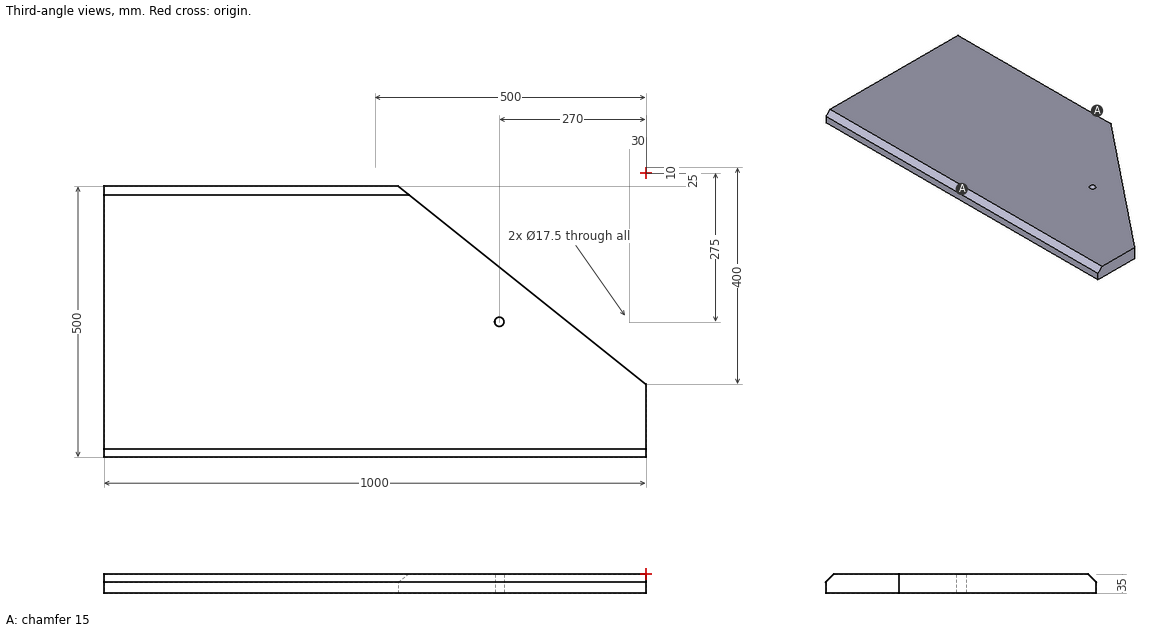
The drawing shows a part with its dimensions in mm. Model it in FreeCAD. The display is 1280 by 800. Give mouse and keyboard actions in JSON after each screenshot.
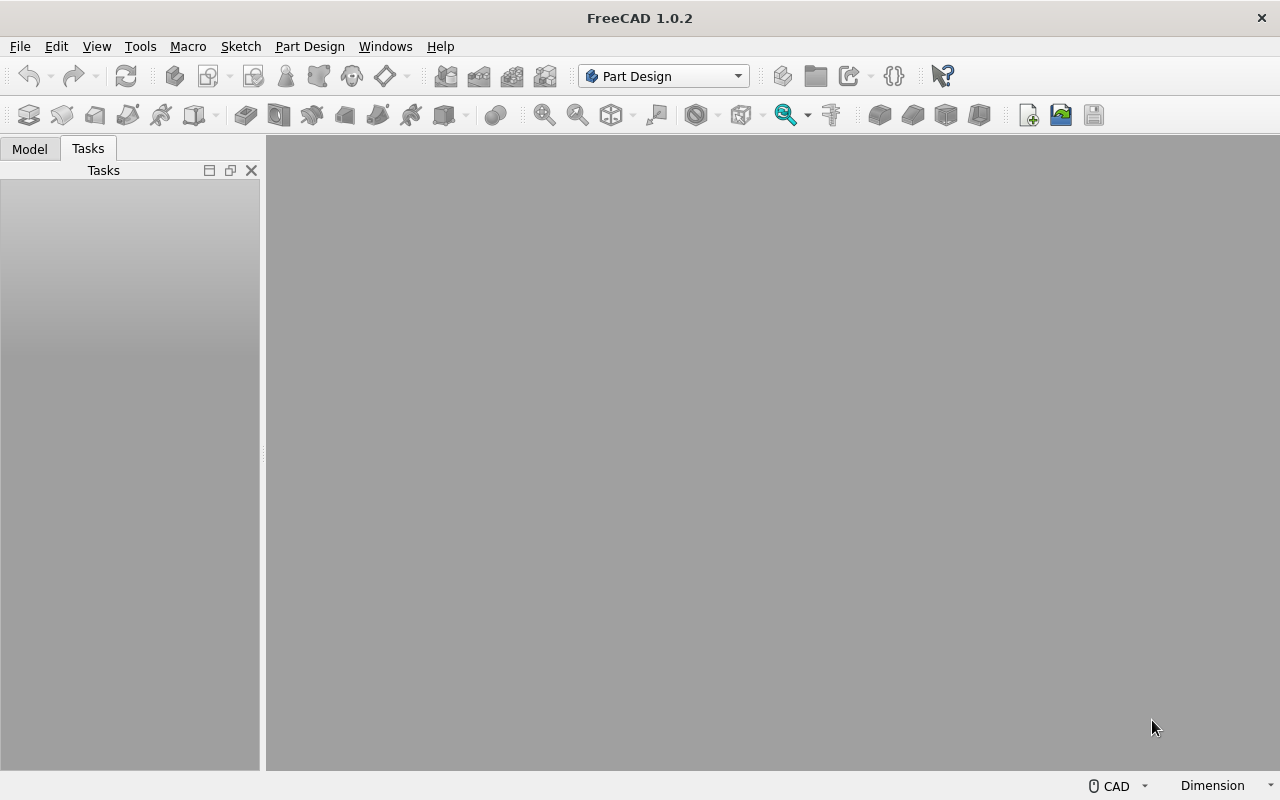
{"action": "key", "text": "ctrl+n"}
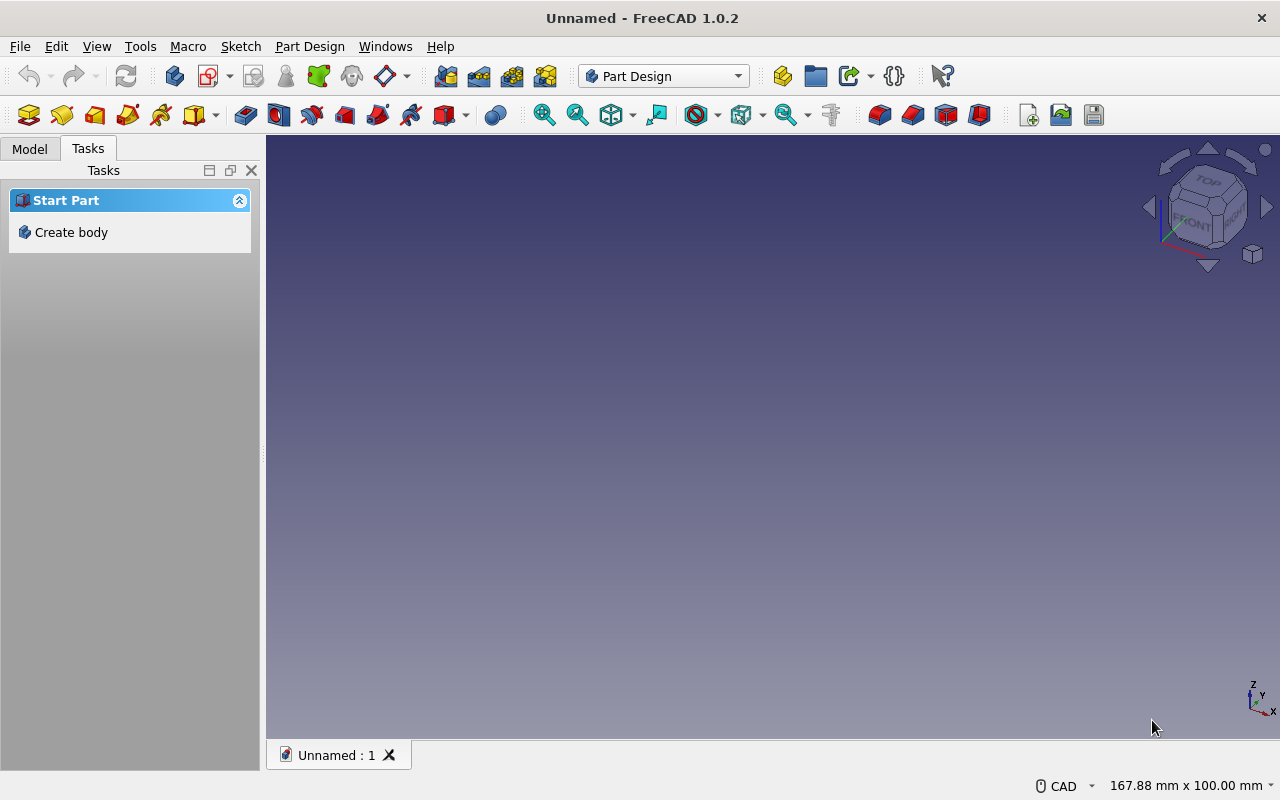
{"action": "left_click", "coordinate": [208, 76]}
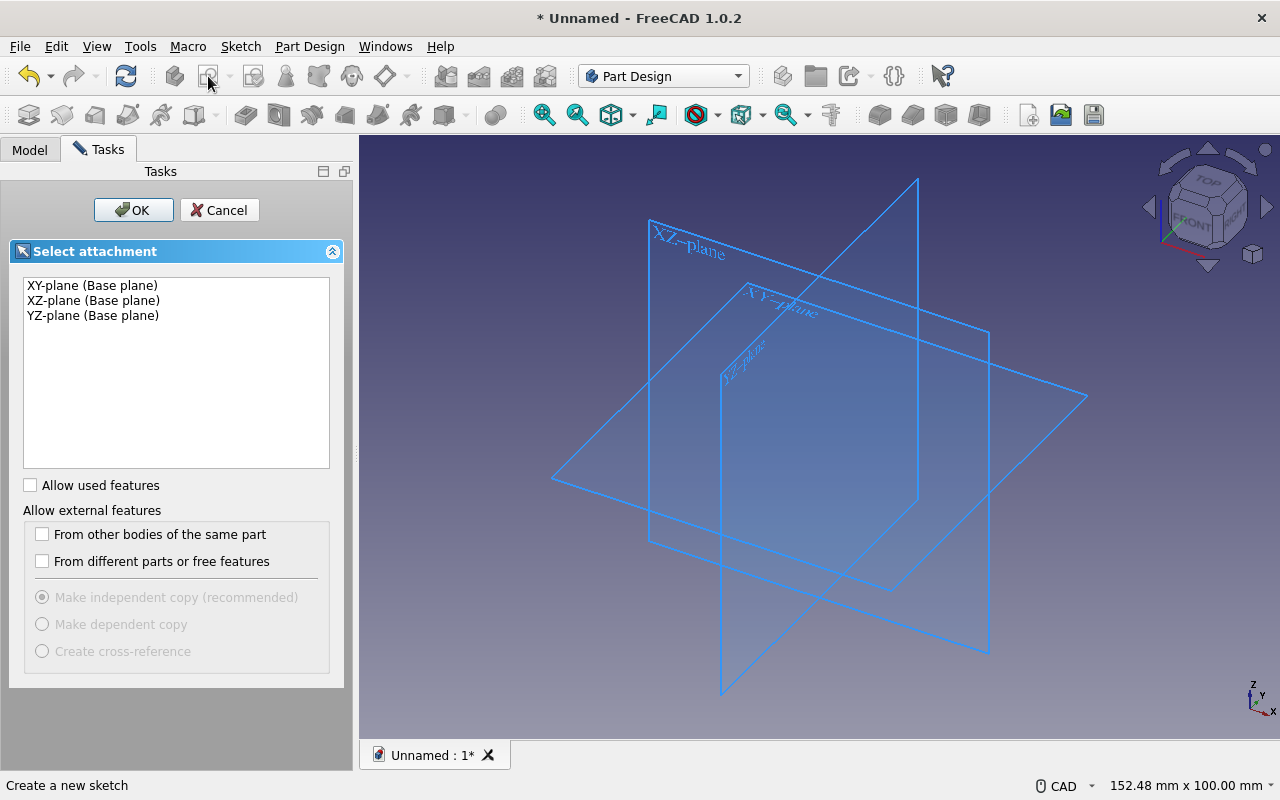
{"action": "left_click", "coordinate": [84, 286]}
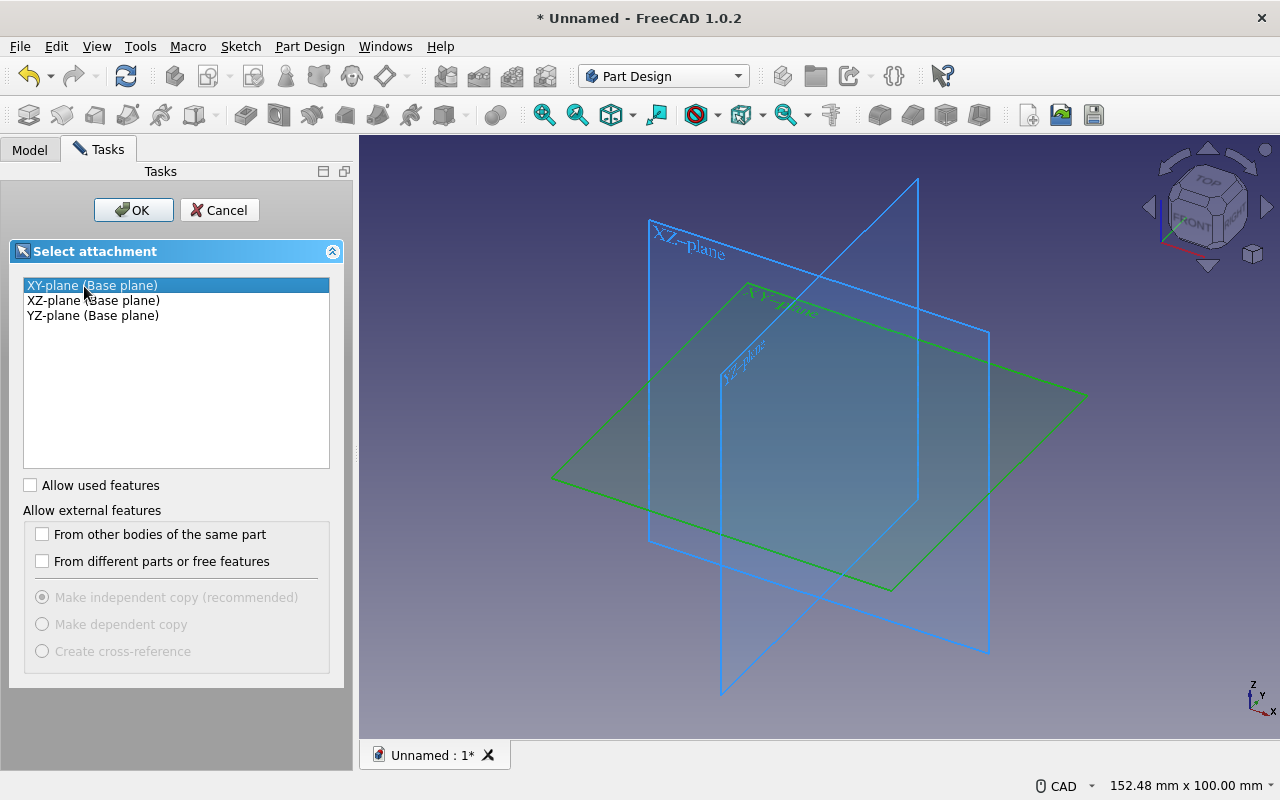
{"action": "left_click", "coordinate": [134, 210]}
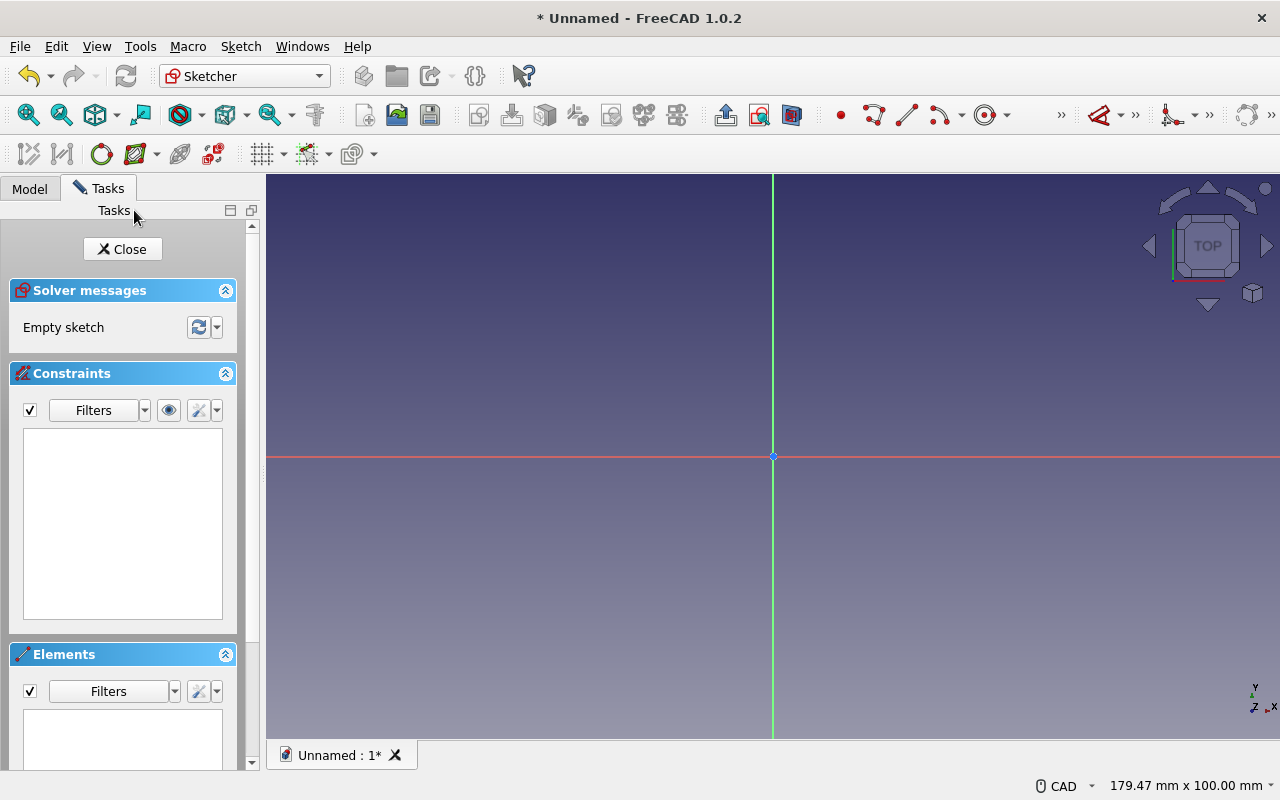
{"action": "scroll", "coordinate": [1048, 272], "scroll_direction": "down", "scroll_amount": 11}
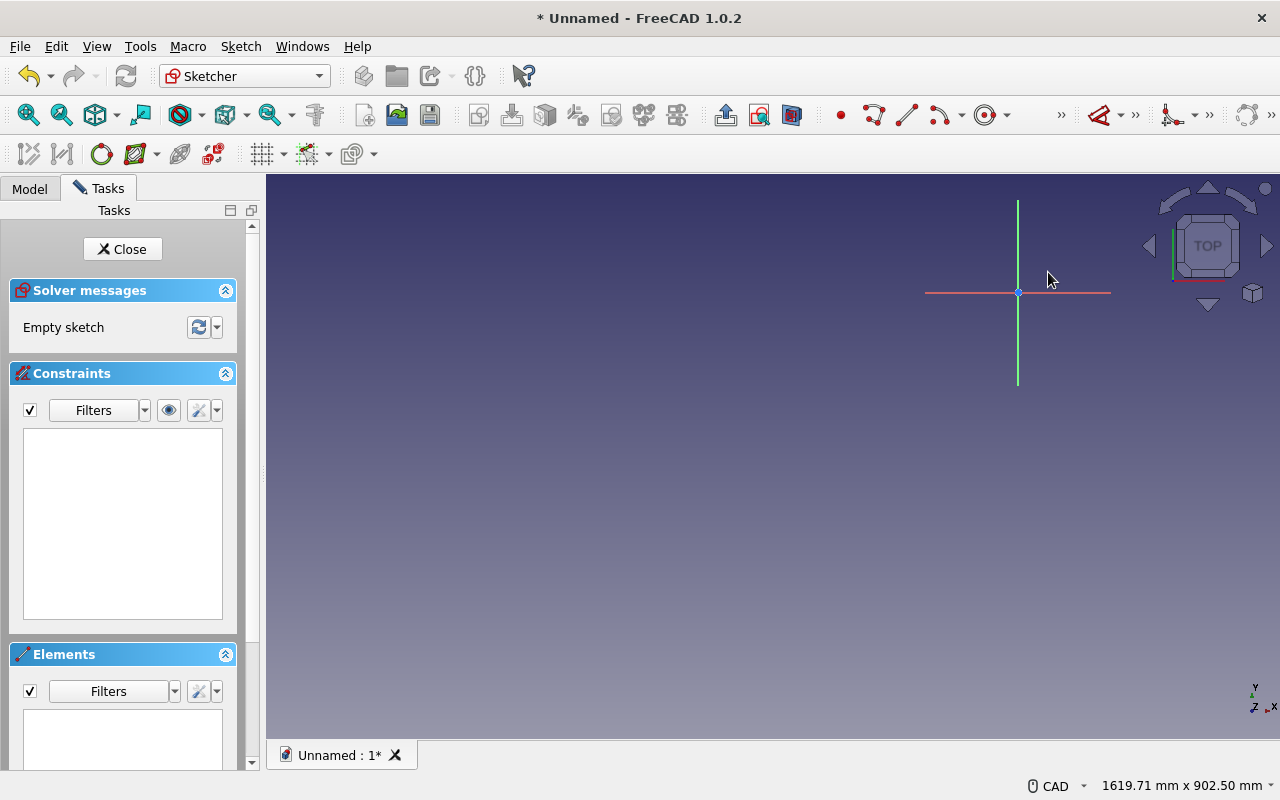
{"action": "key", "text": "g r"}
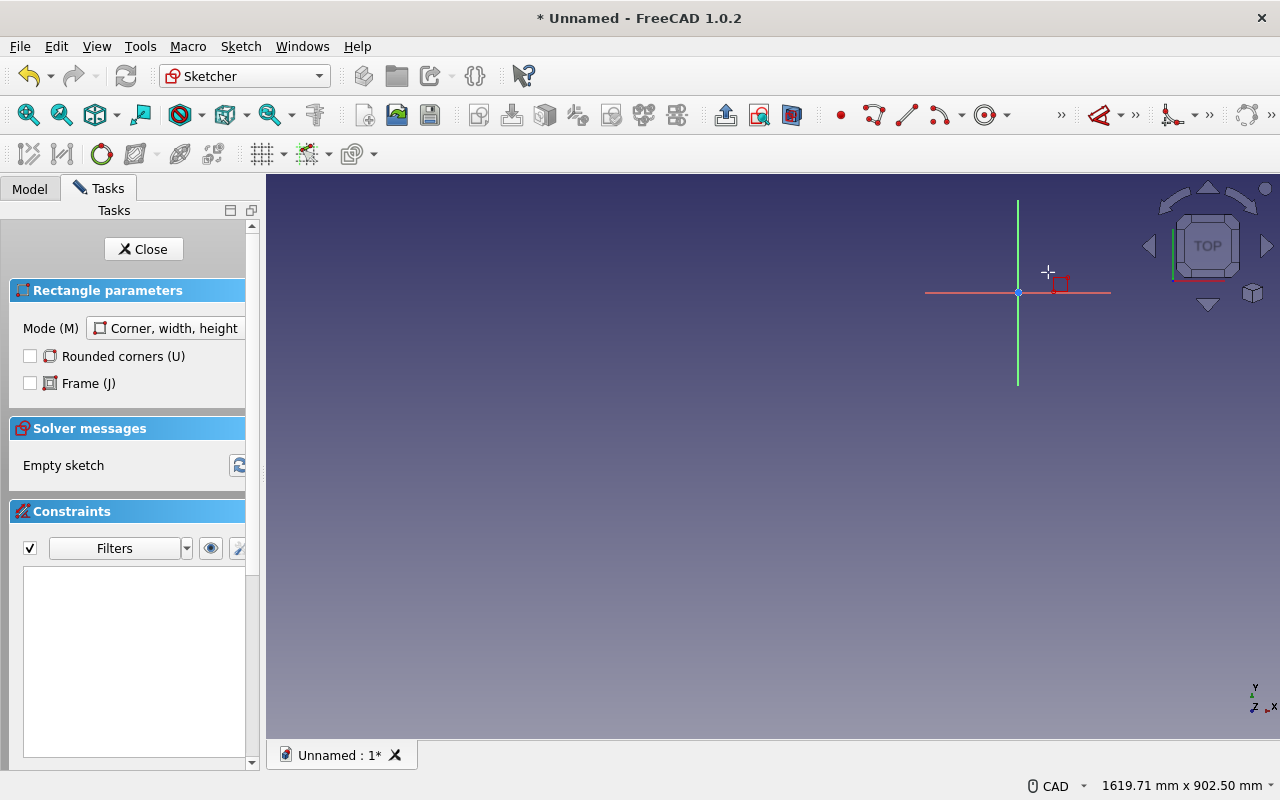
{"action": "left_click", "coordinate": [392, 308]}
{"action": "left_click", "coordinate": [1018, 621]}
{"action": "key", "text": "Escape"}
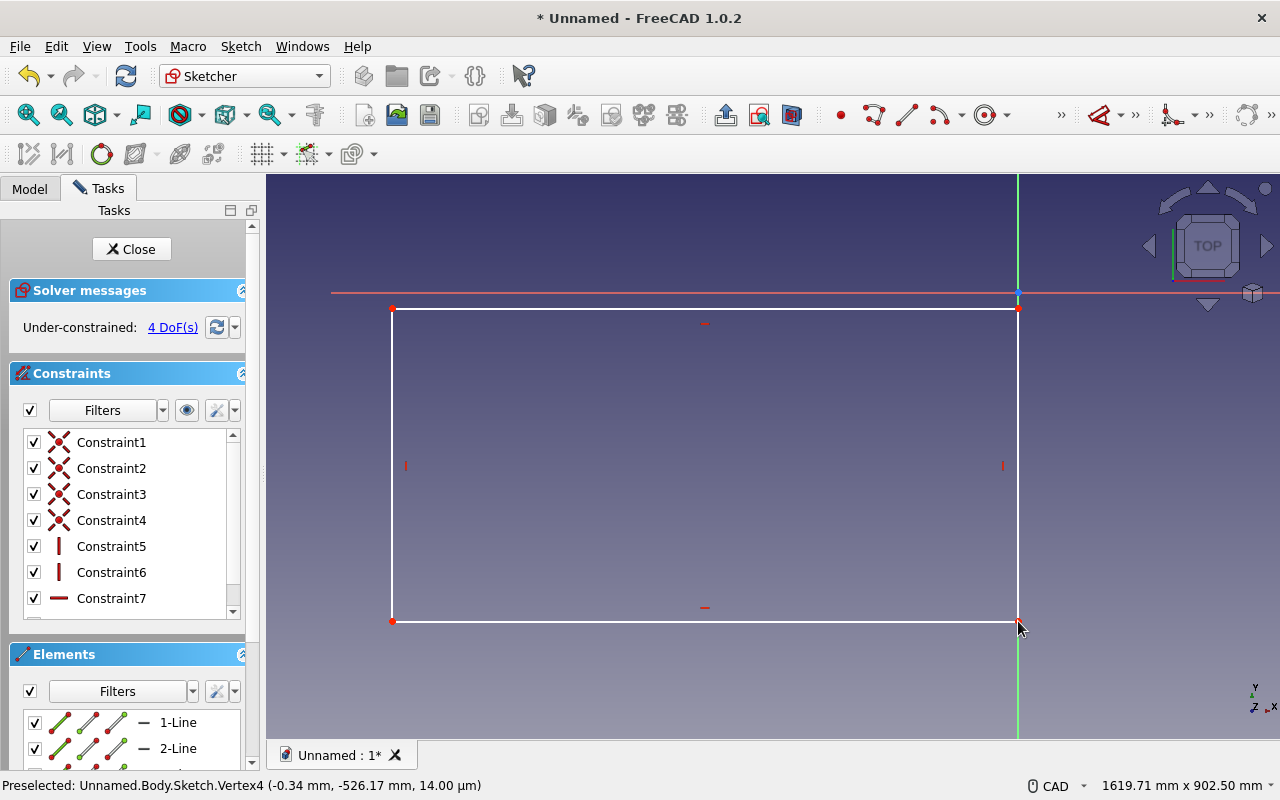
{"action": "left_click", "coordinate": [1018, 622]}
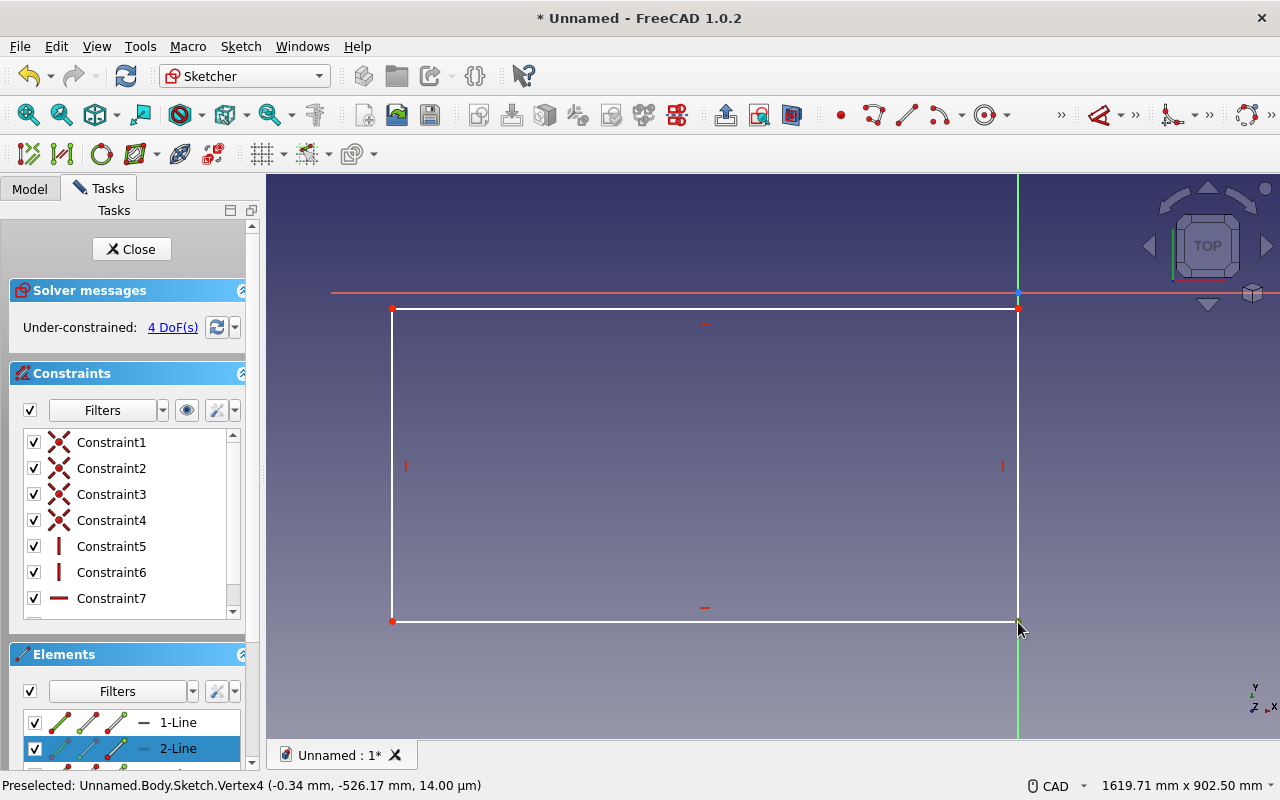
{"action": "left_click", "coordinate": [1018, 675]}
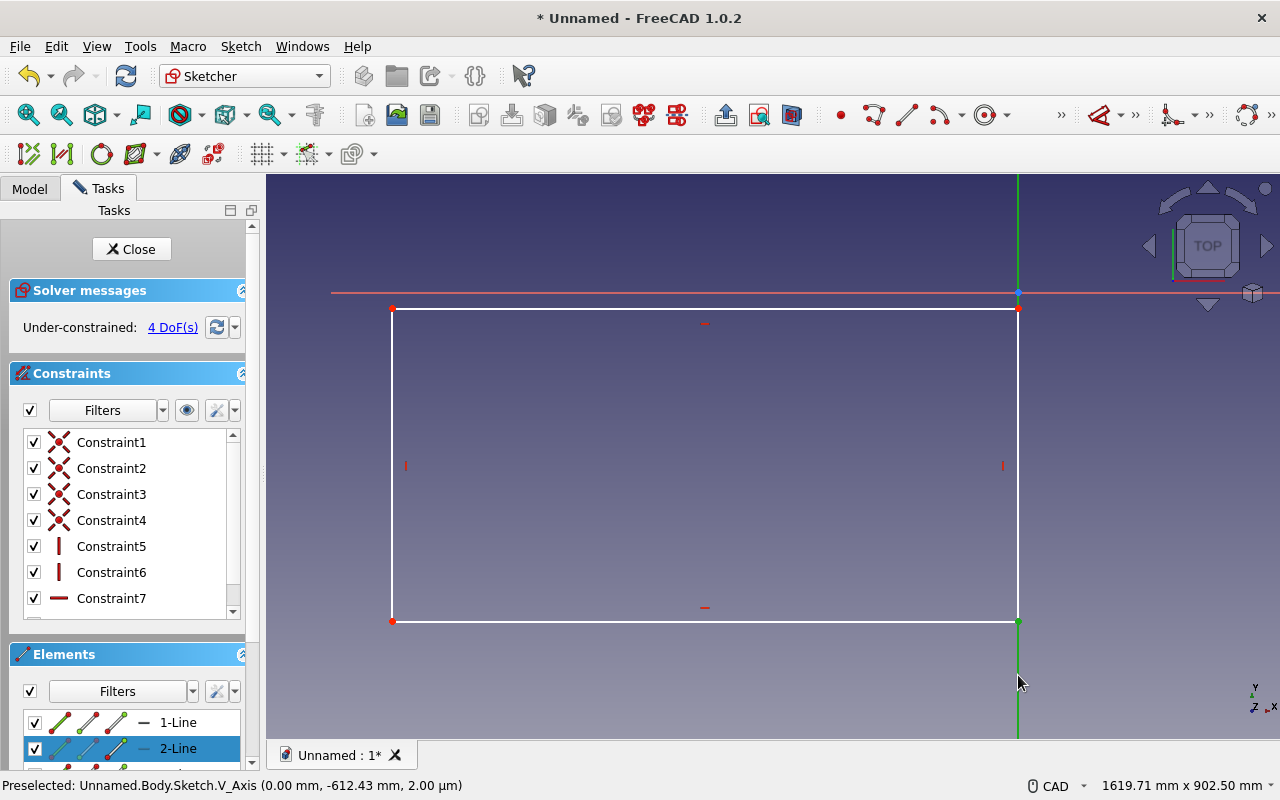
{"action": "key", "text": "c"}